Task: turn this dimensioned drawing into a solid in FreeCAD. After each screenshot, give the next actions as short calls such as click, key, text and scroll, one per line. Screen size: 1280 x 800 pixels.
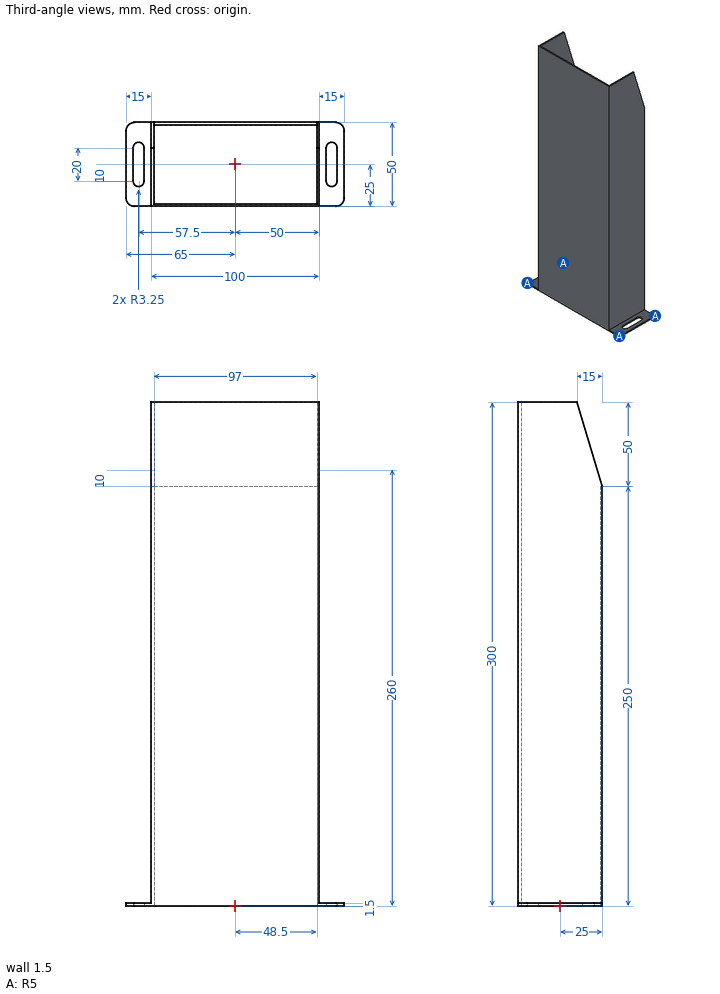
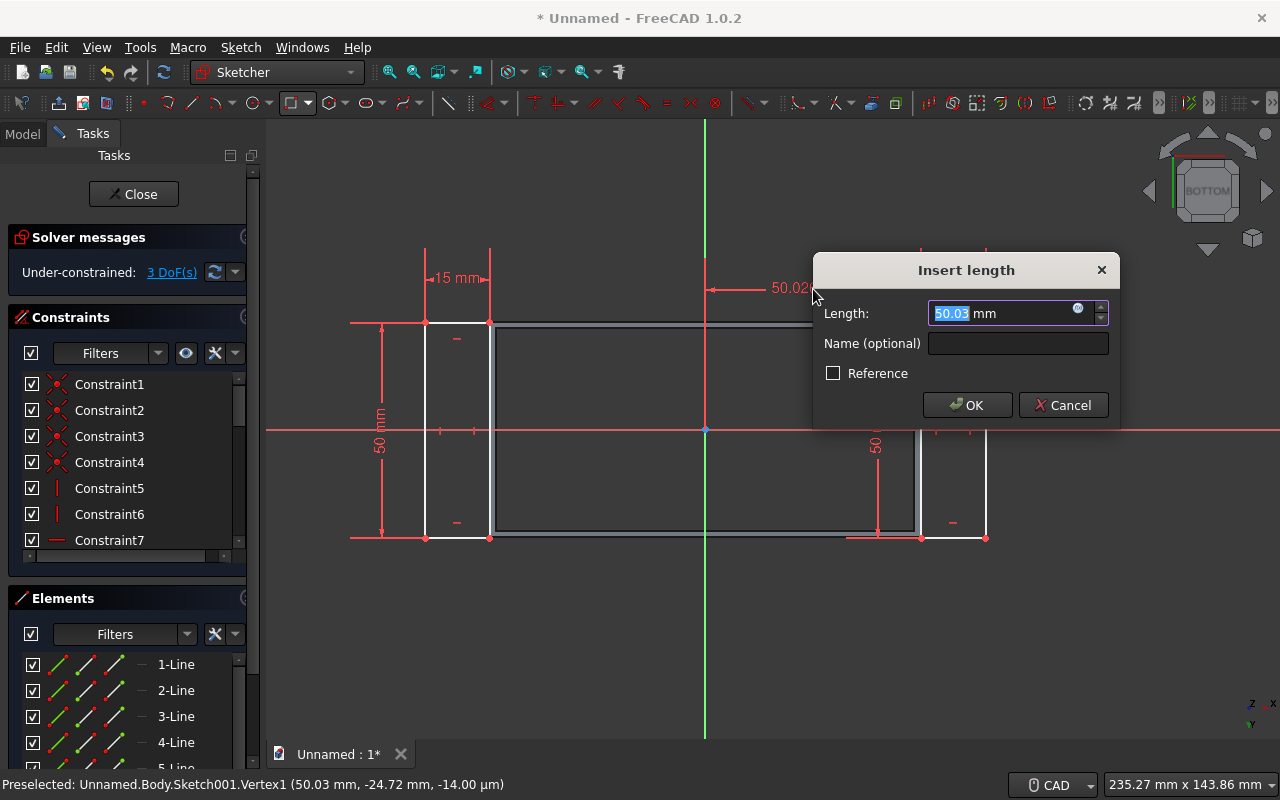
text(50)
key(Return)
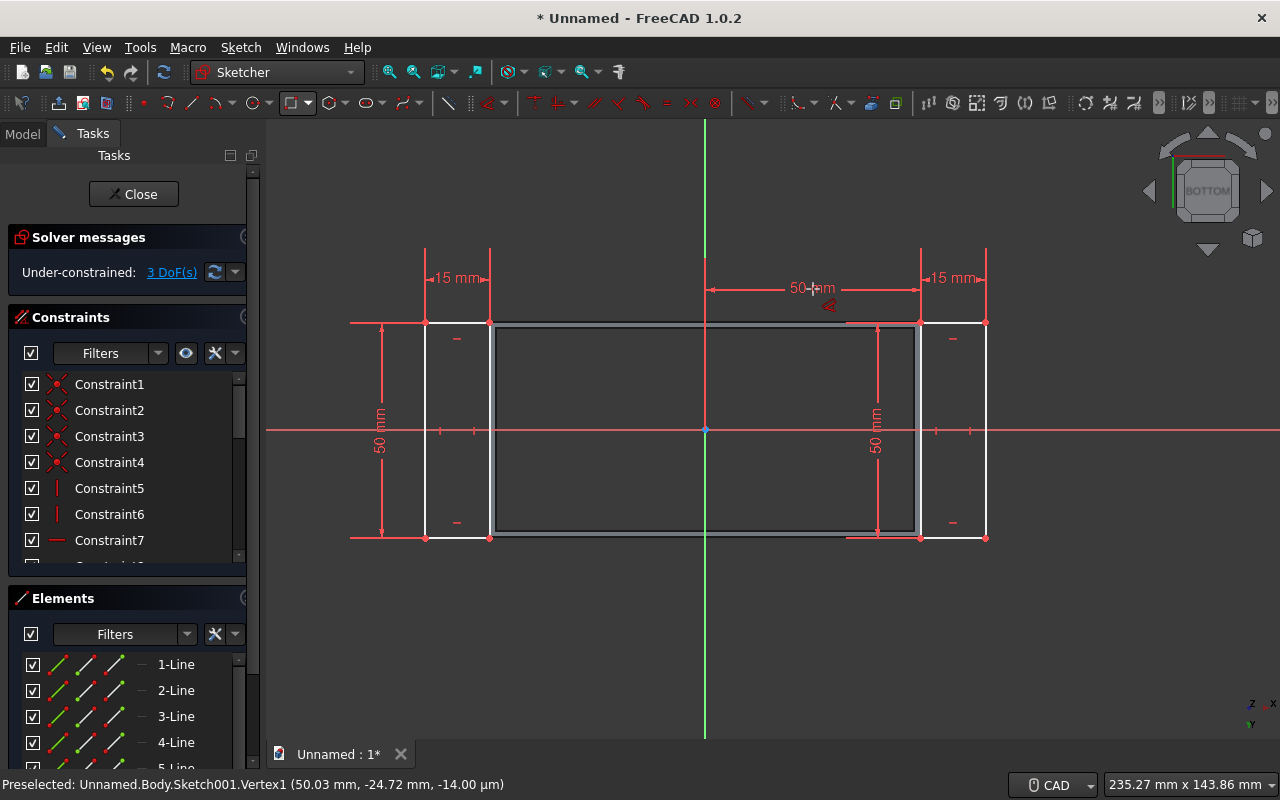
click(921, 323)
click(955, 376)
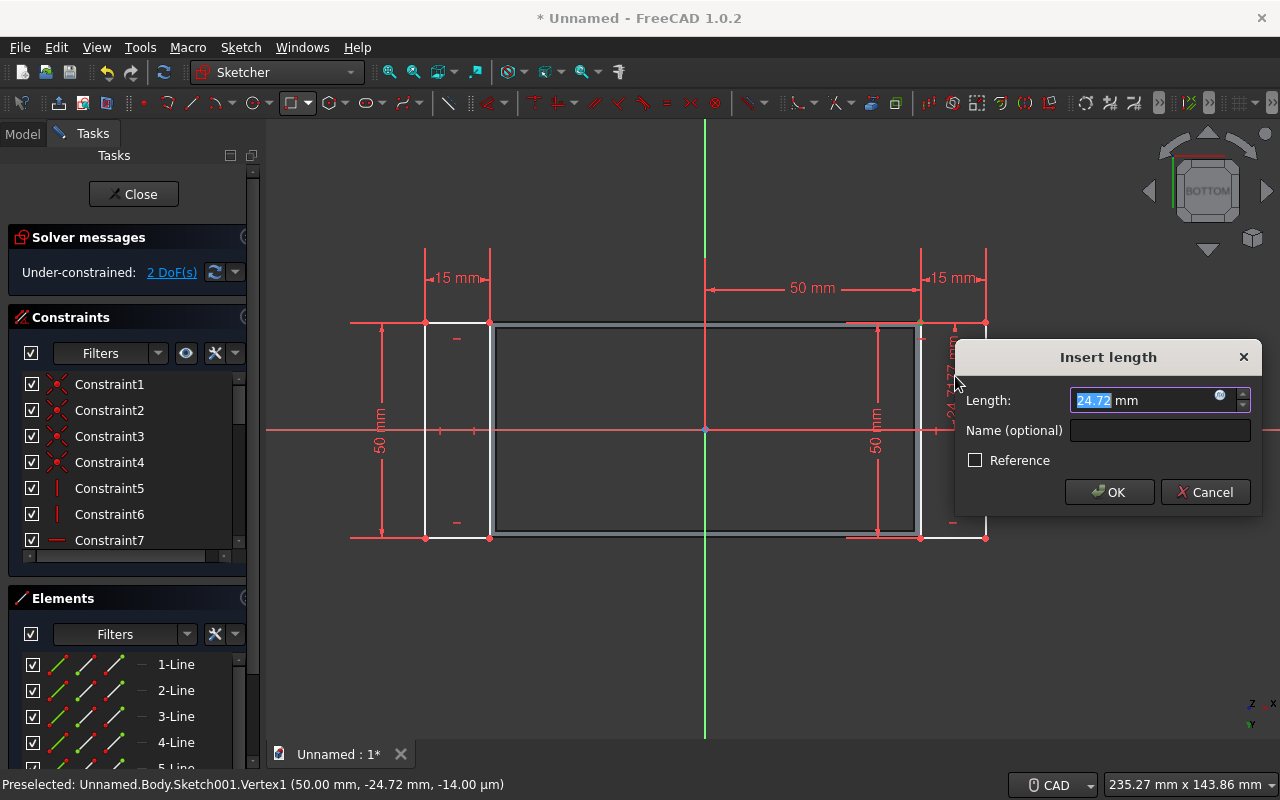
text(25)
key(Return)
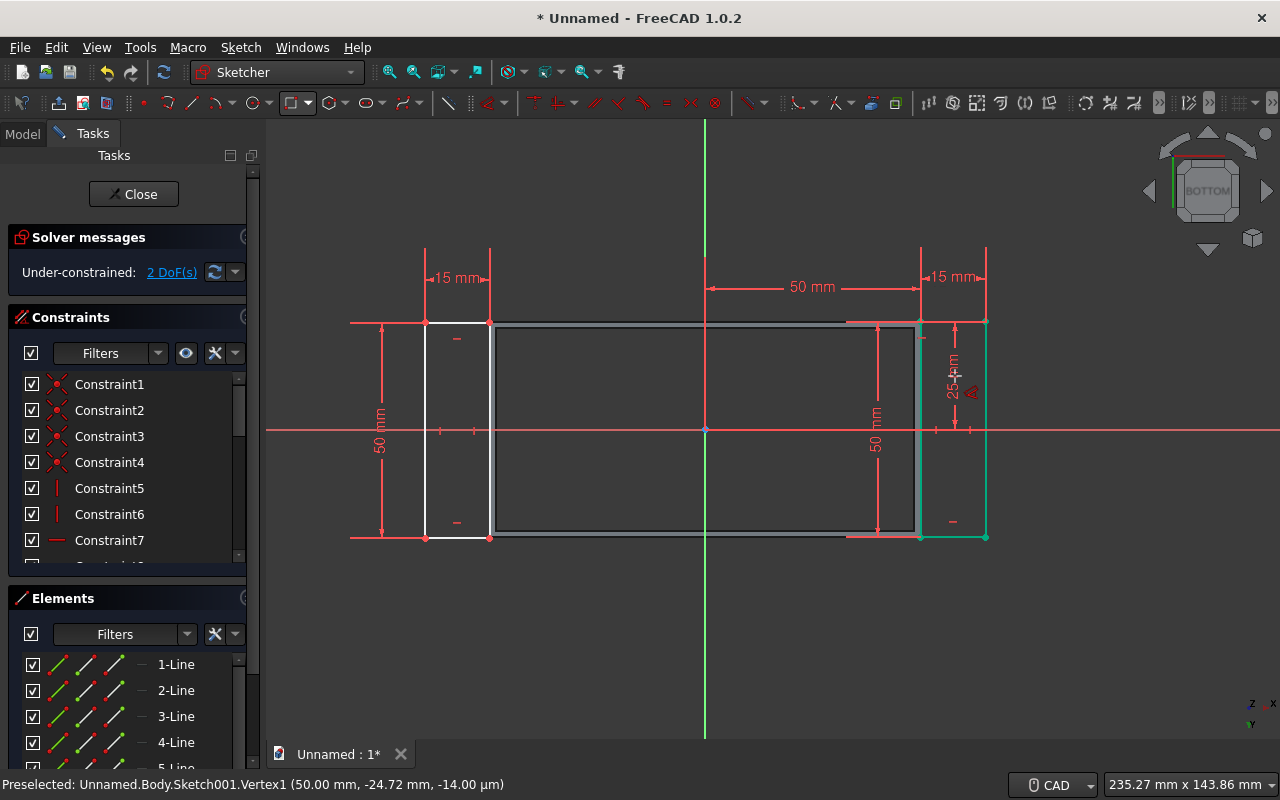
click(425, 323)
click(565, 289)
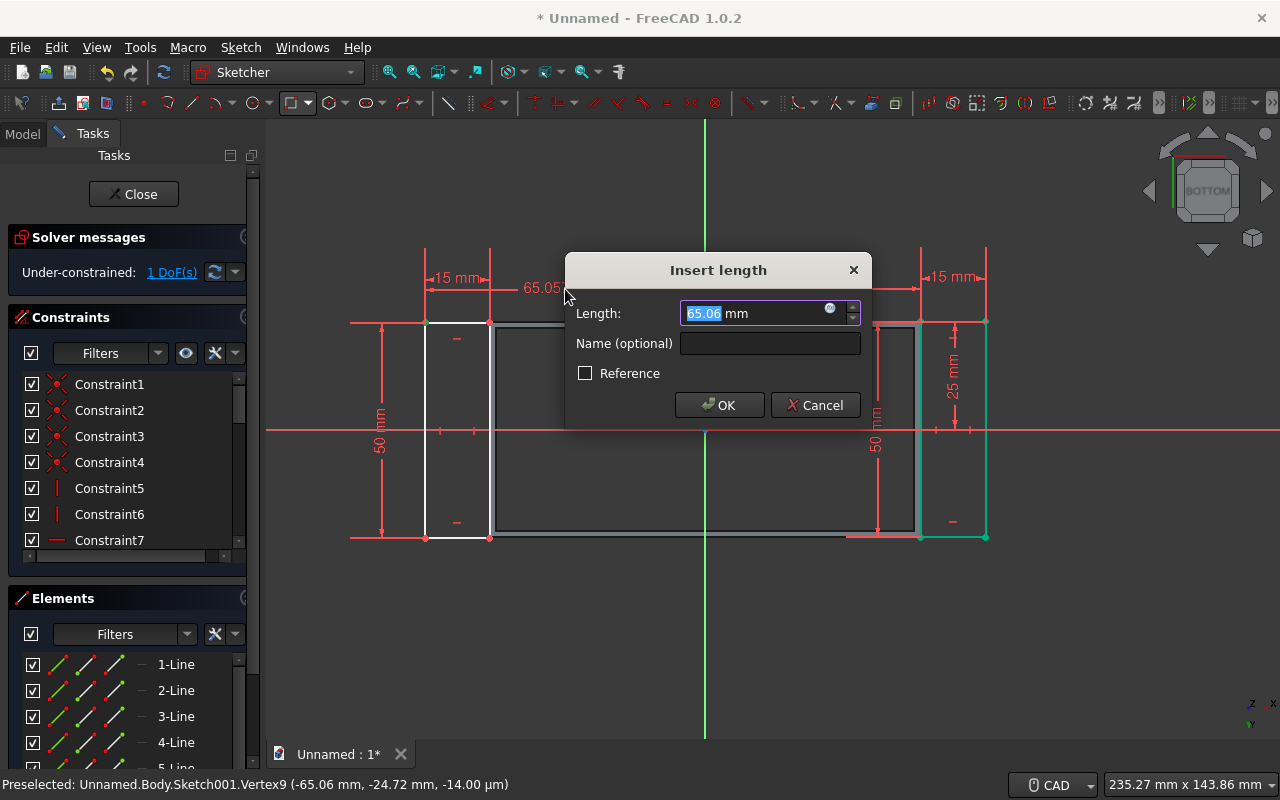
text(65)
key(Return)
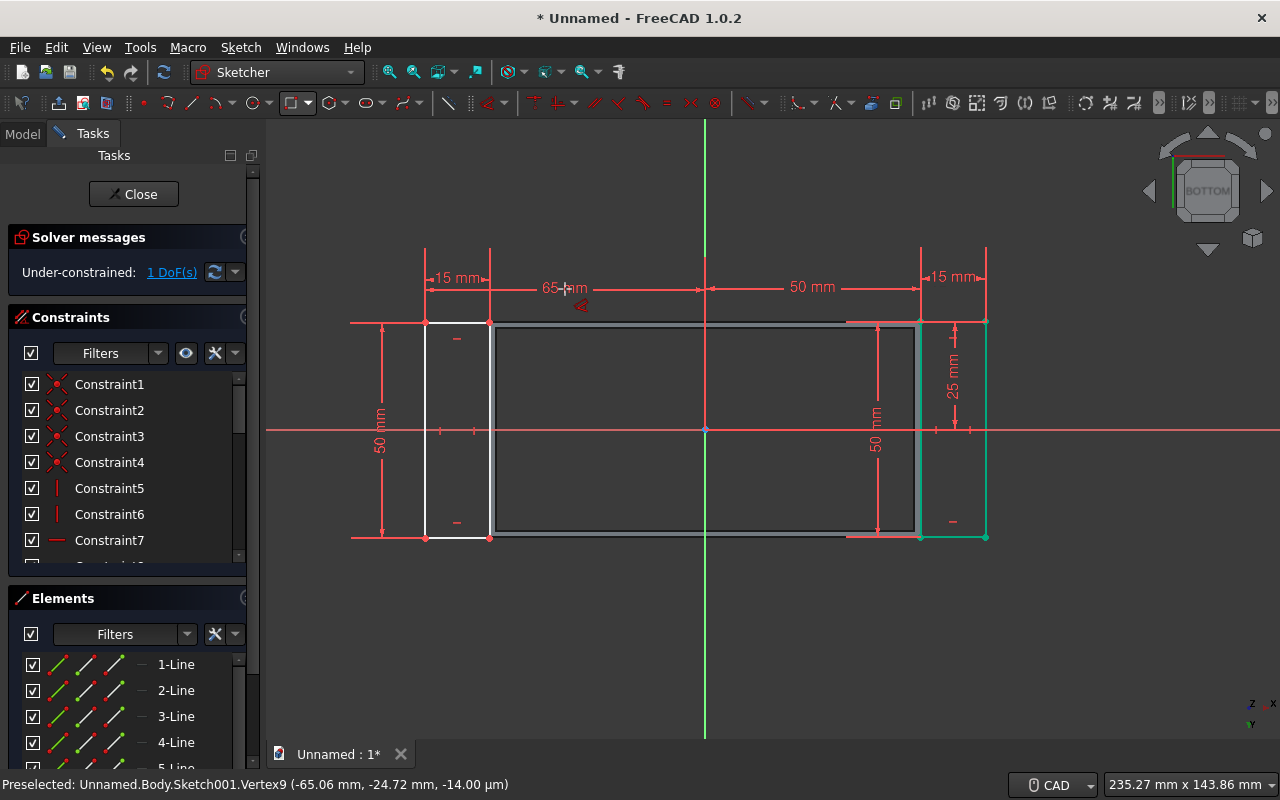
click(425, 323)
click(391, 376)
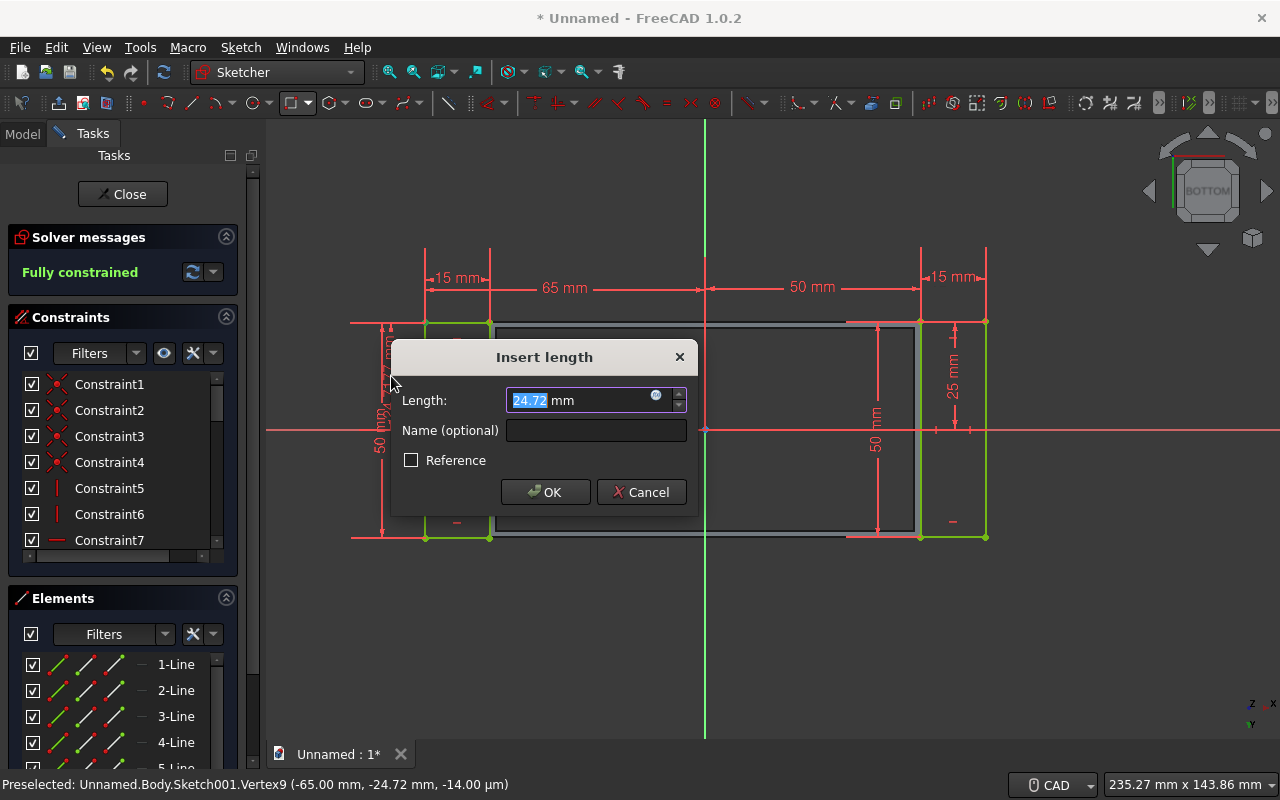
text(25)
key(Return)
key(Escape)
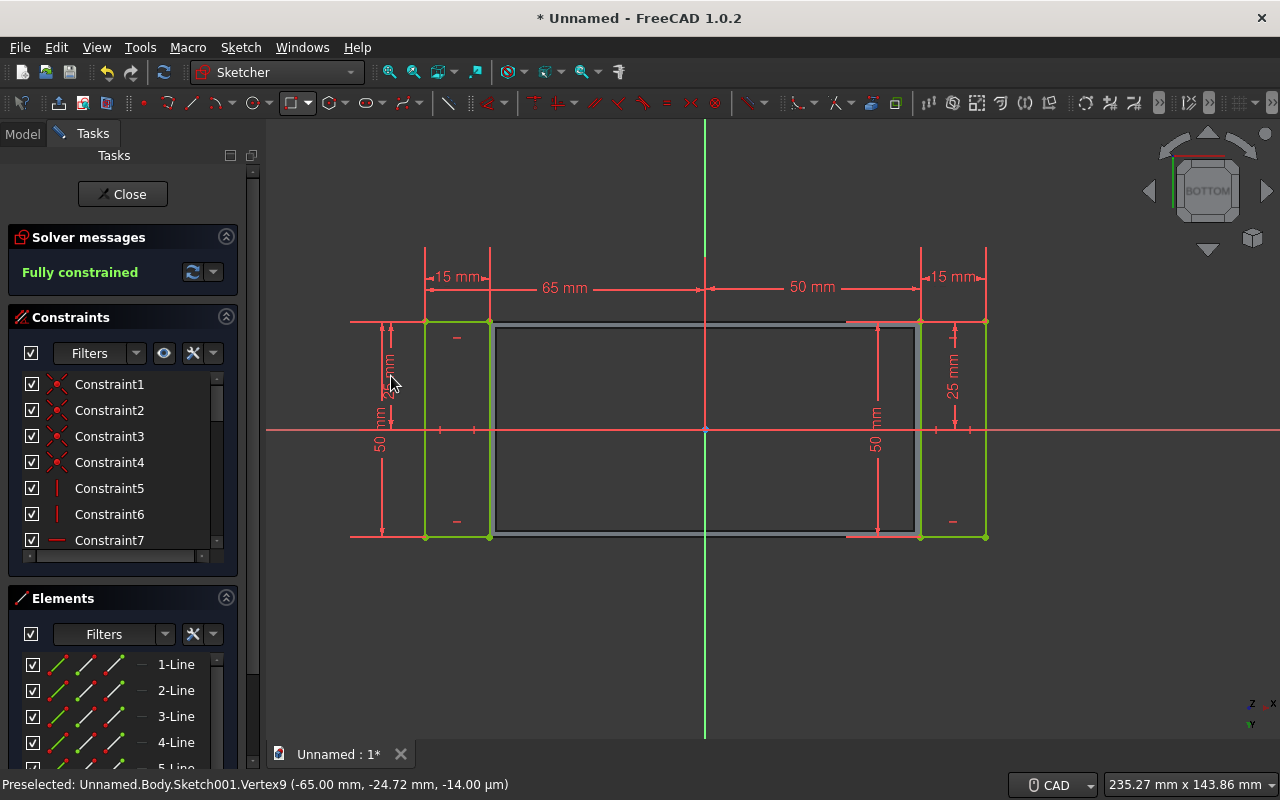
click(123, 194)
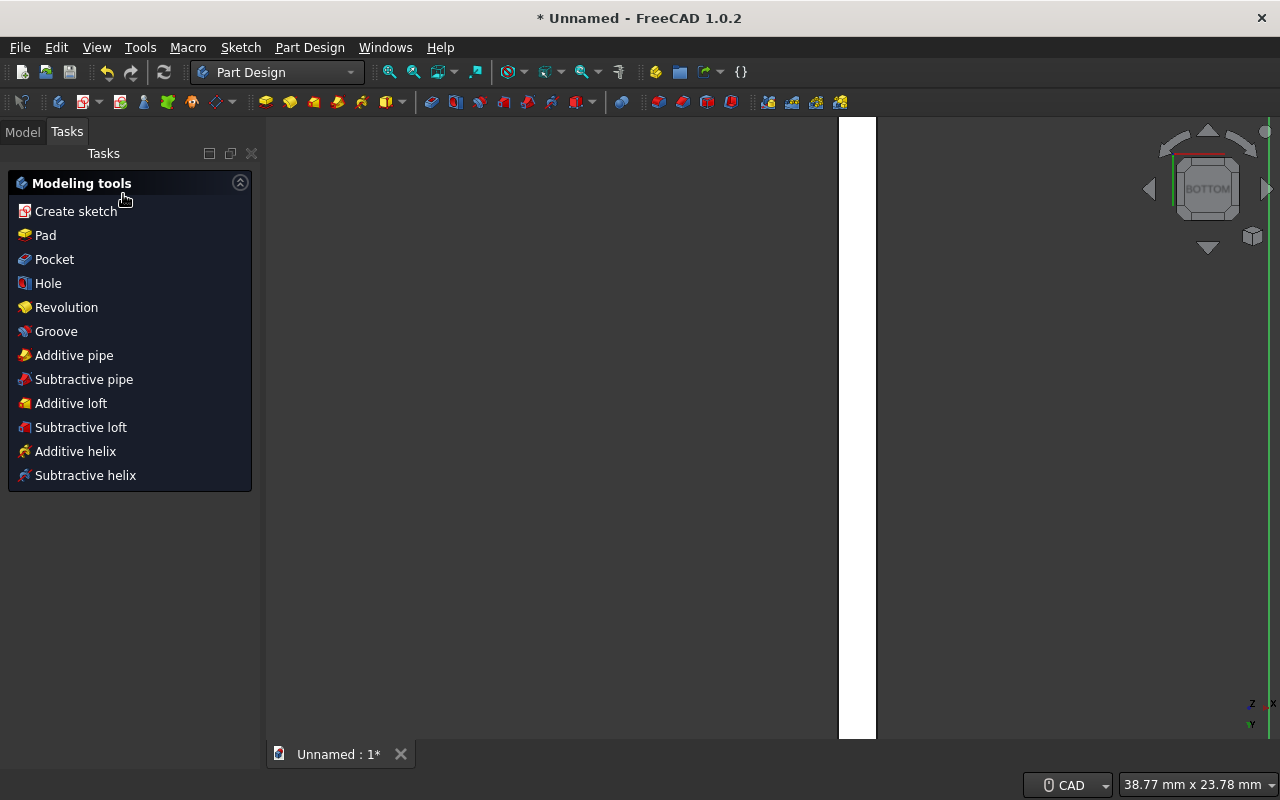
click(266, 102)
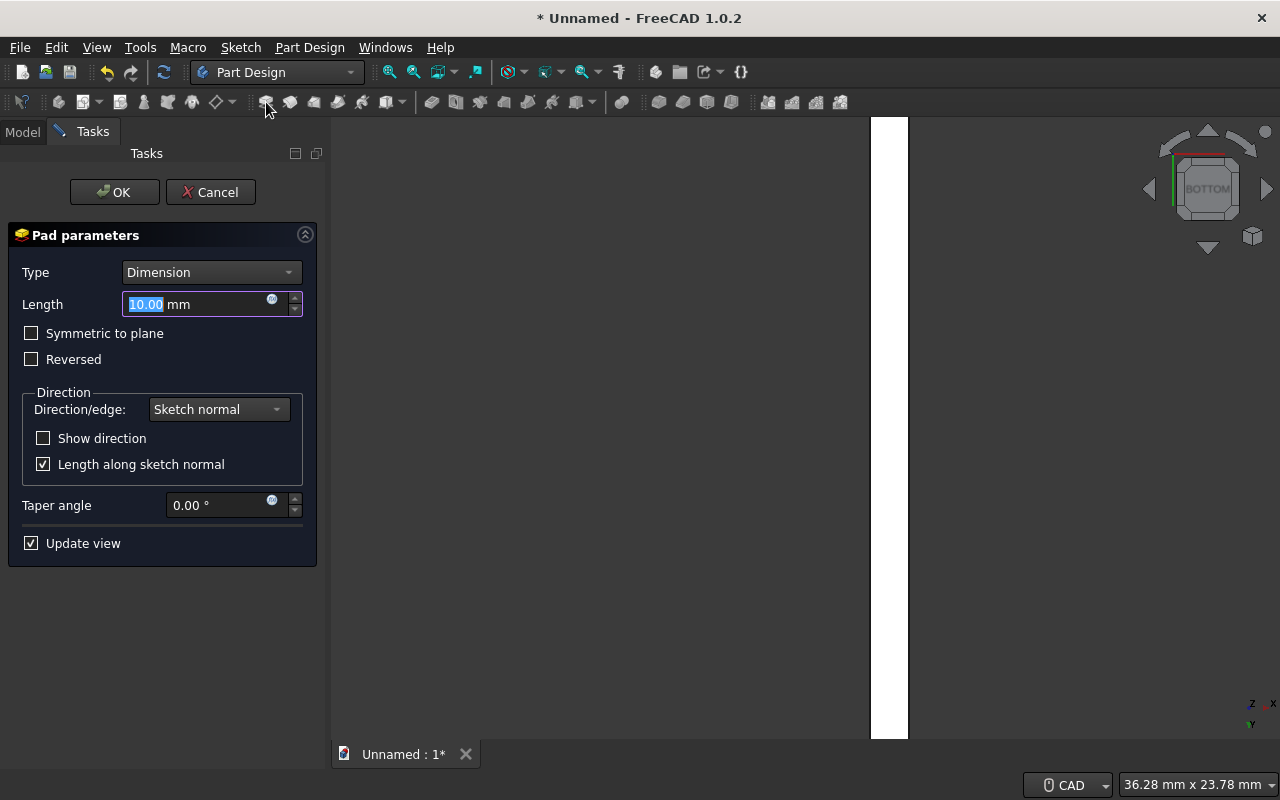
text(1.5)
key(Tab)